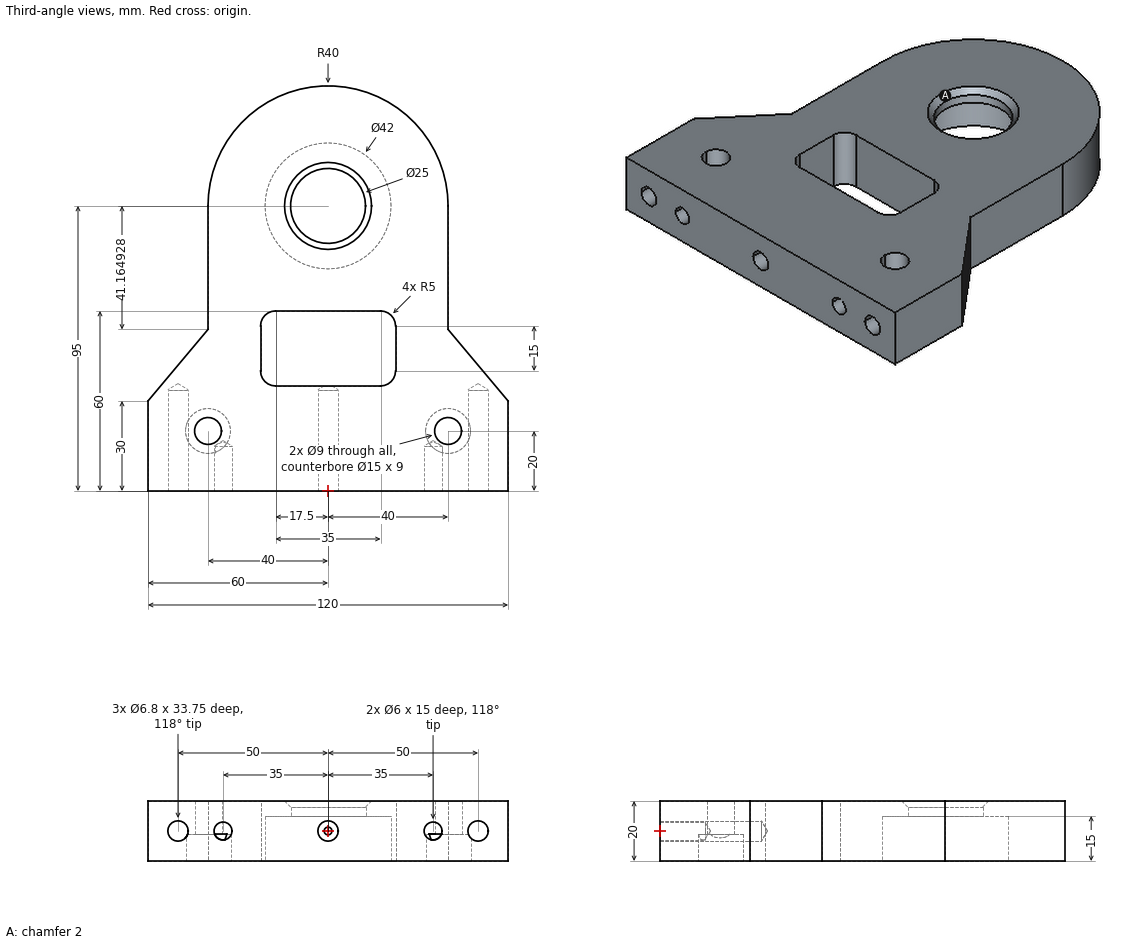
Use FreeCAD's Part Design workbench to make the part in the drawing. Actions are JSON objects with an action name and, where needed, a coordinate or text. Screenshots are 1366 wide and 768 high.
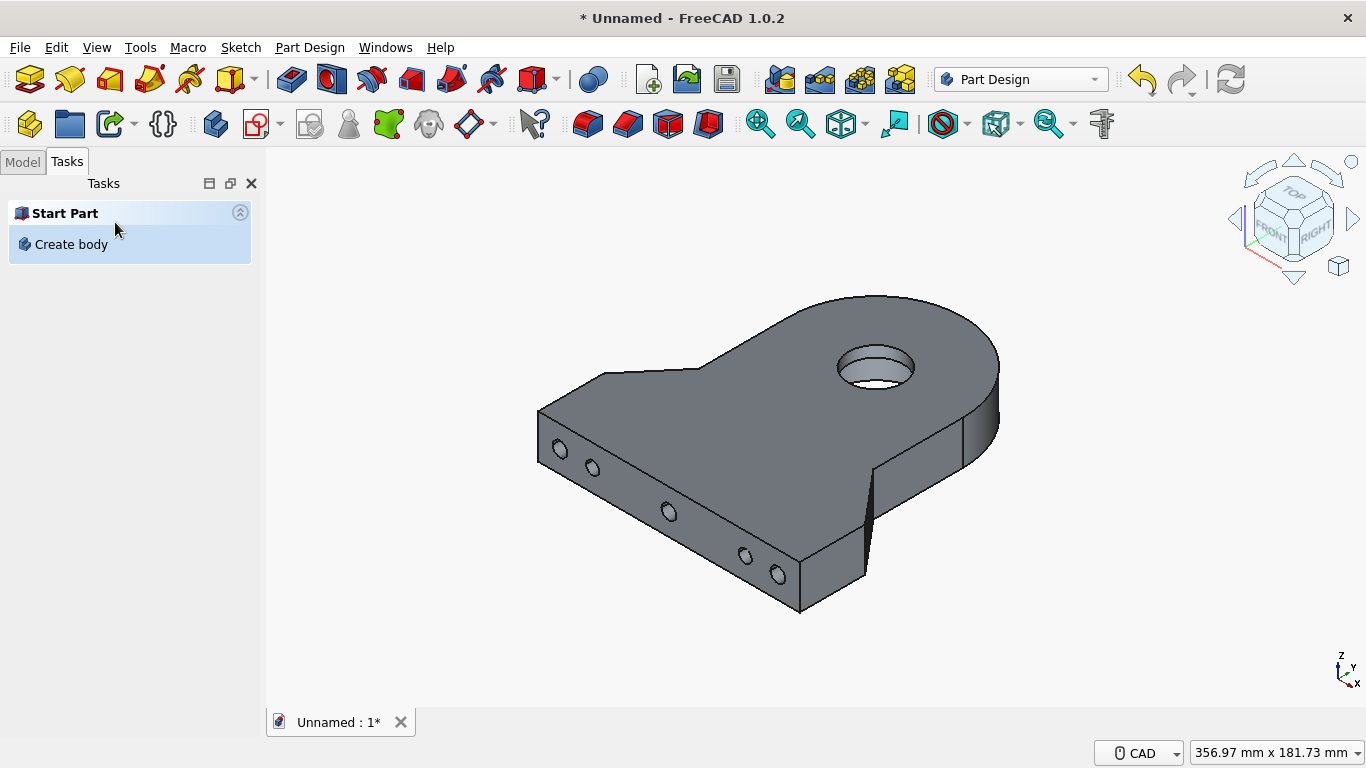
{"action": "left_click", "coordinate": [849, 351]}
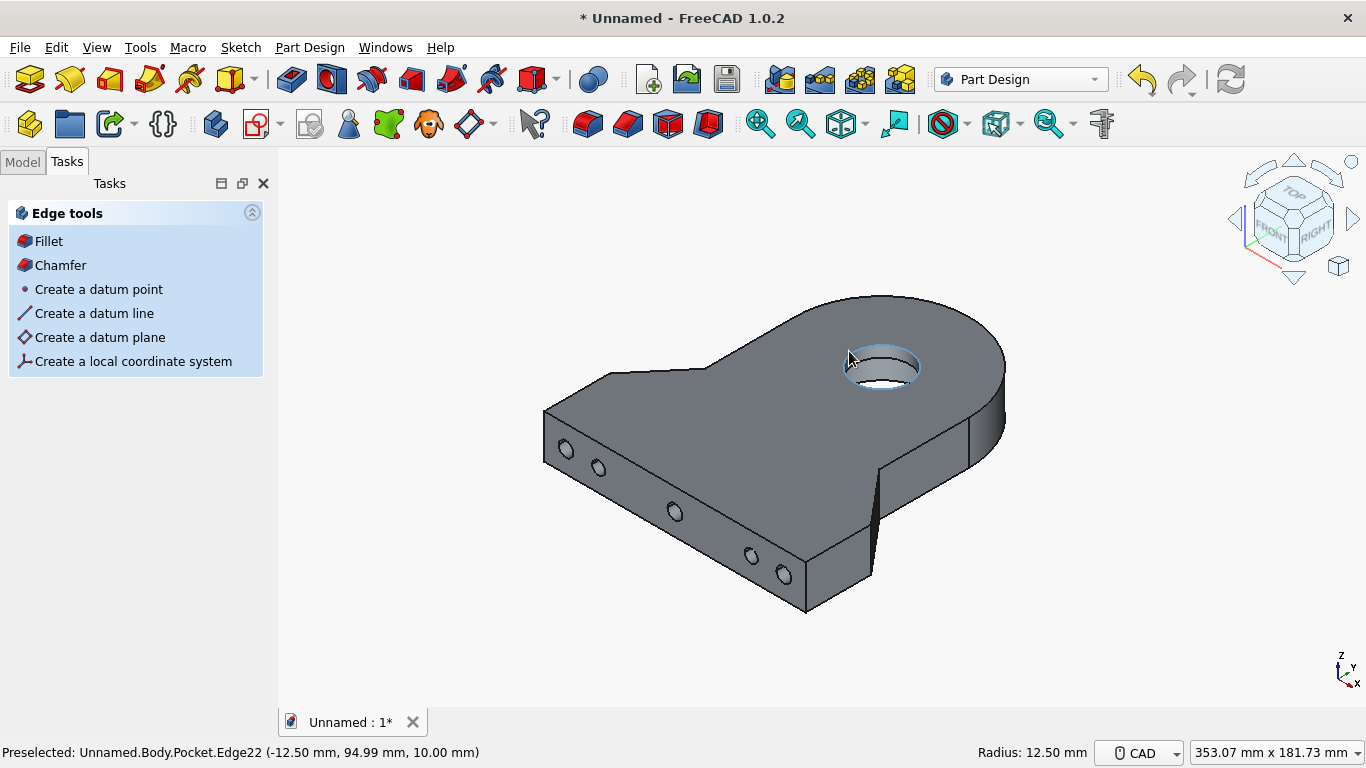
{"action": "left_click", "coordinate": [628, 124]}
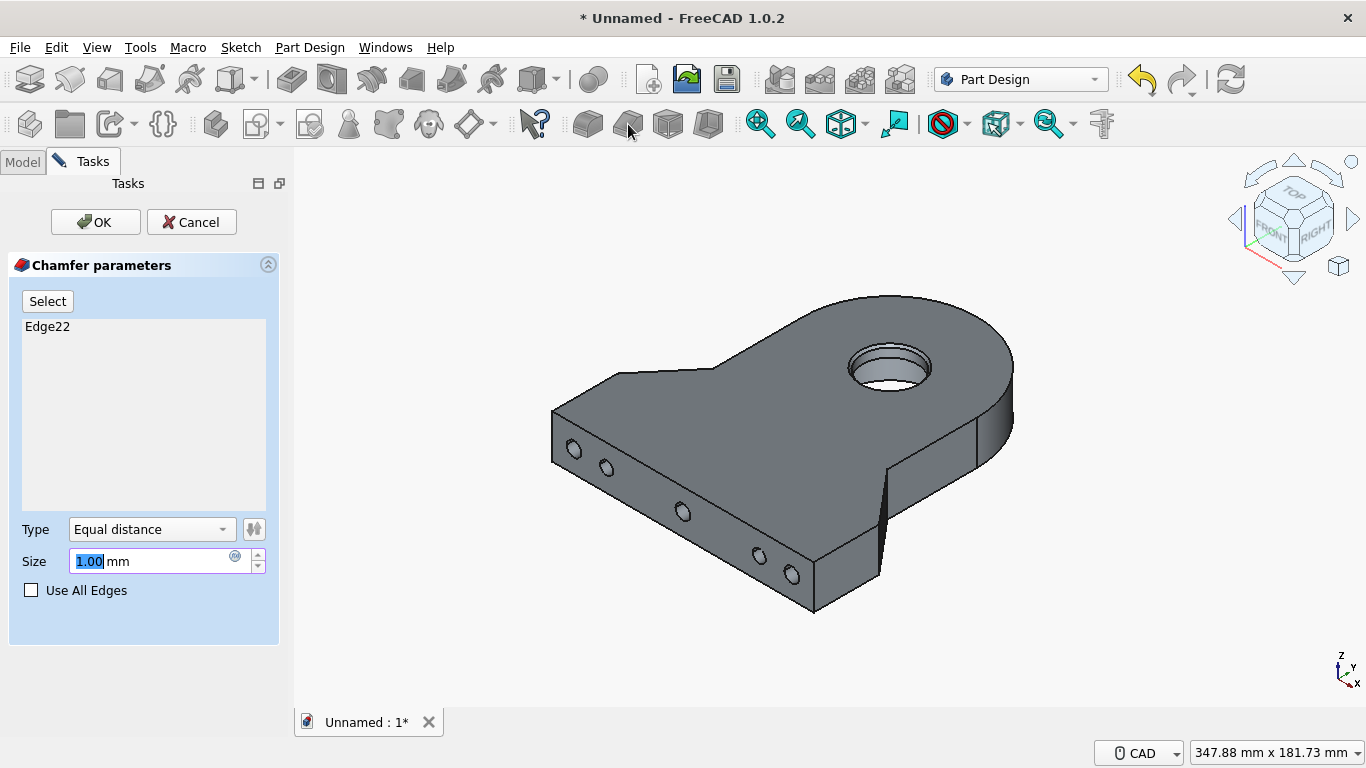
{"action": "type", "text": "2"}
{"action": "key", "text": "Tab"}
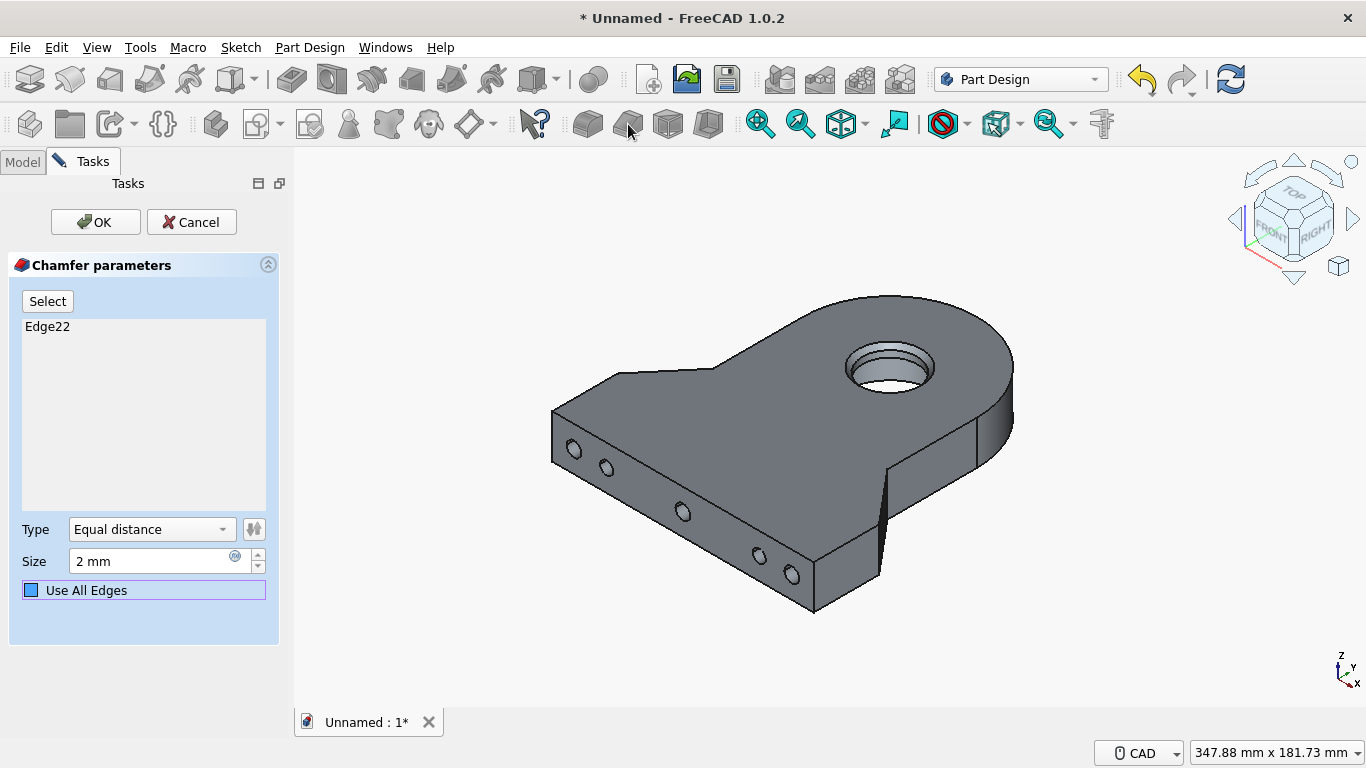
{"action": "left_click", "coordinate": [96, 222]}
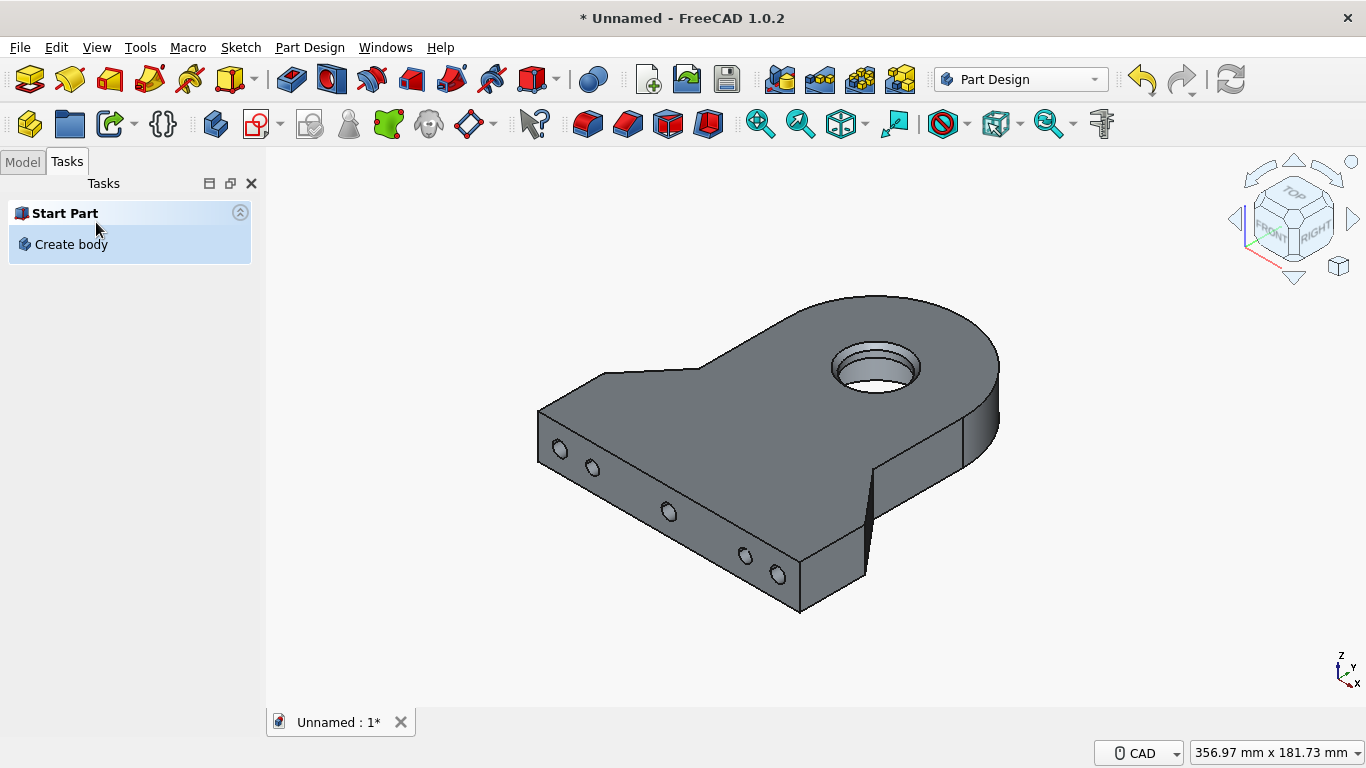
{"action": "key", "text": "5"}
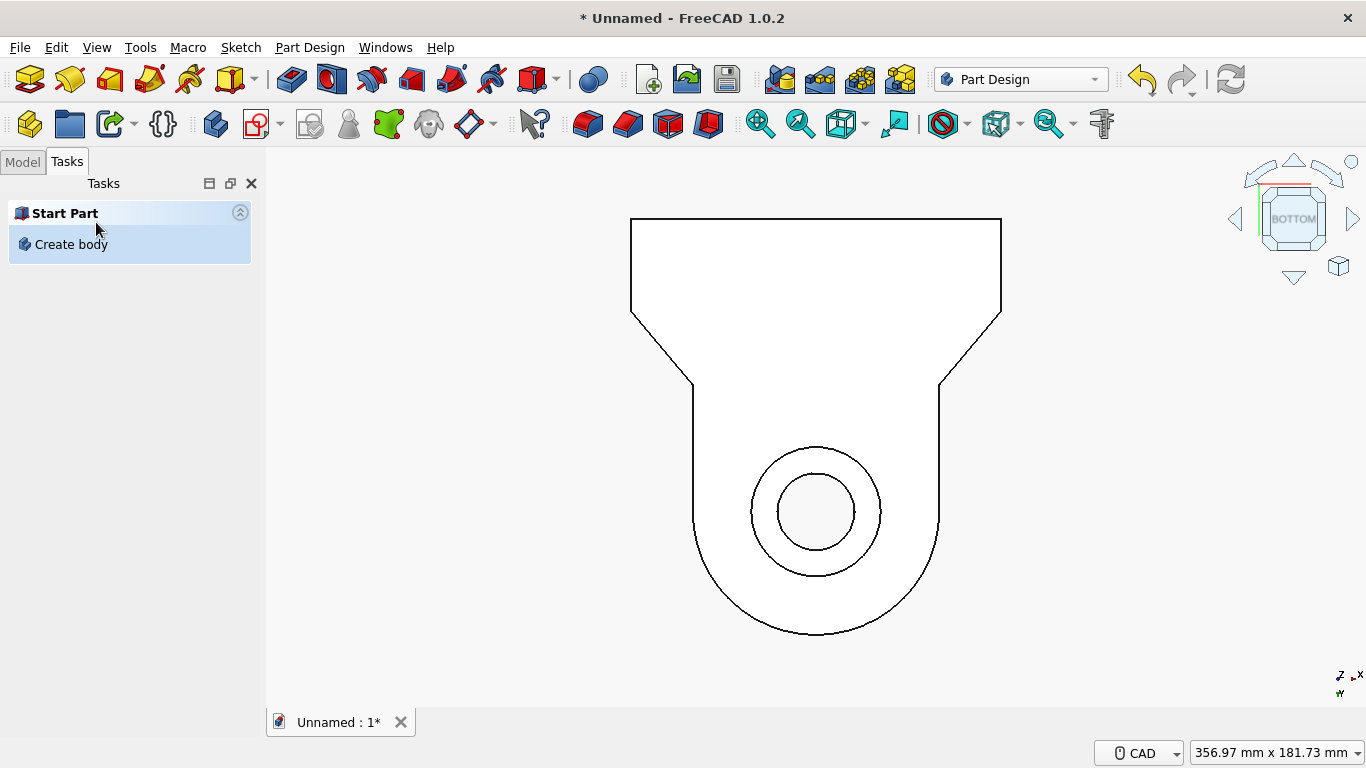
{"action": "left_click", "coordinate": [869, 307]}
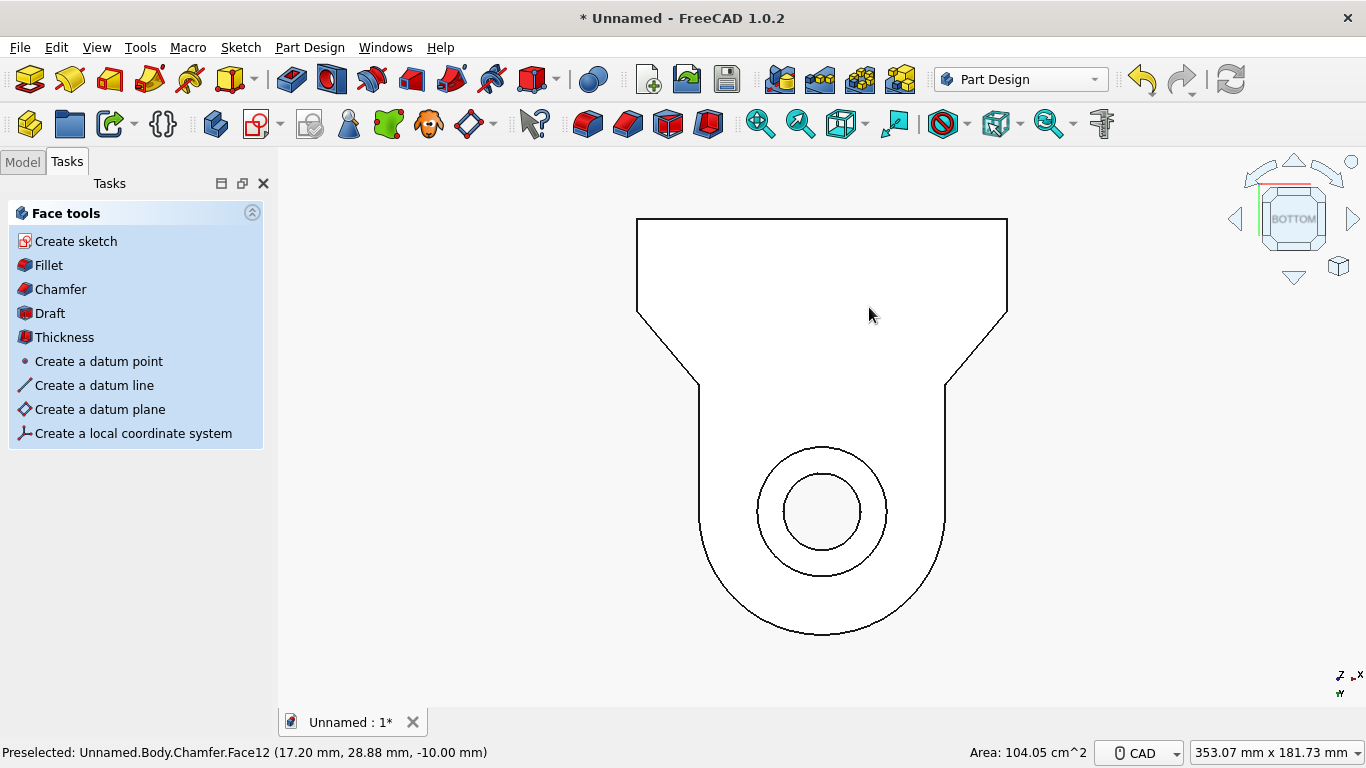
{"action": "left_click", "coordinate": [256, 124]}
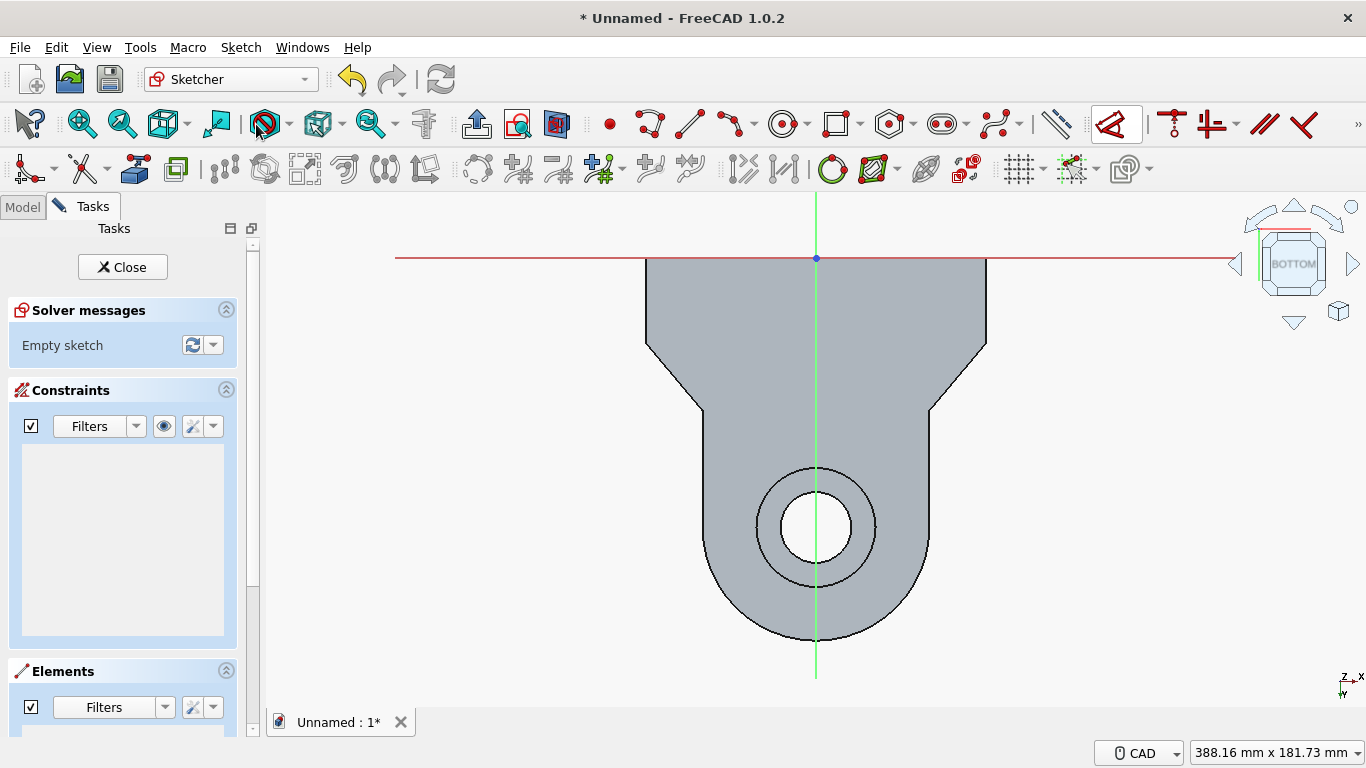
{"action": "scroll", "coordinate": [856, 220], "scroll_direction": "up", "scroll_amount": 5}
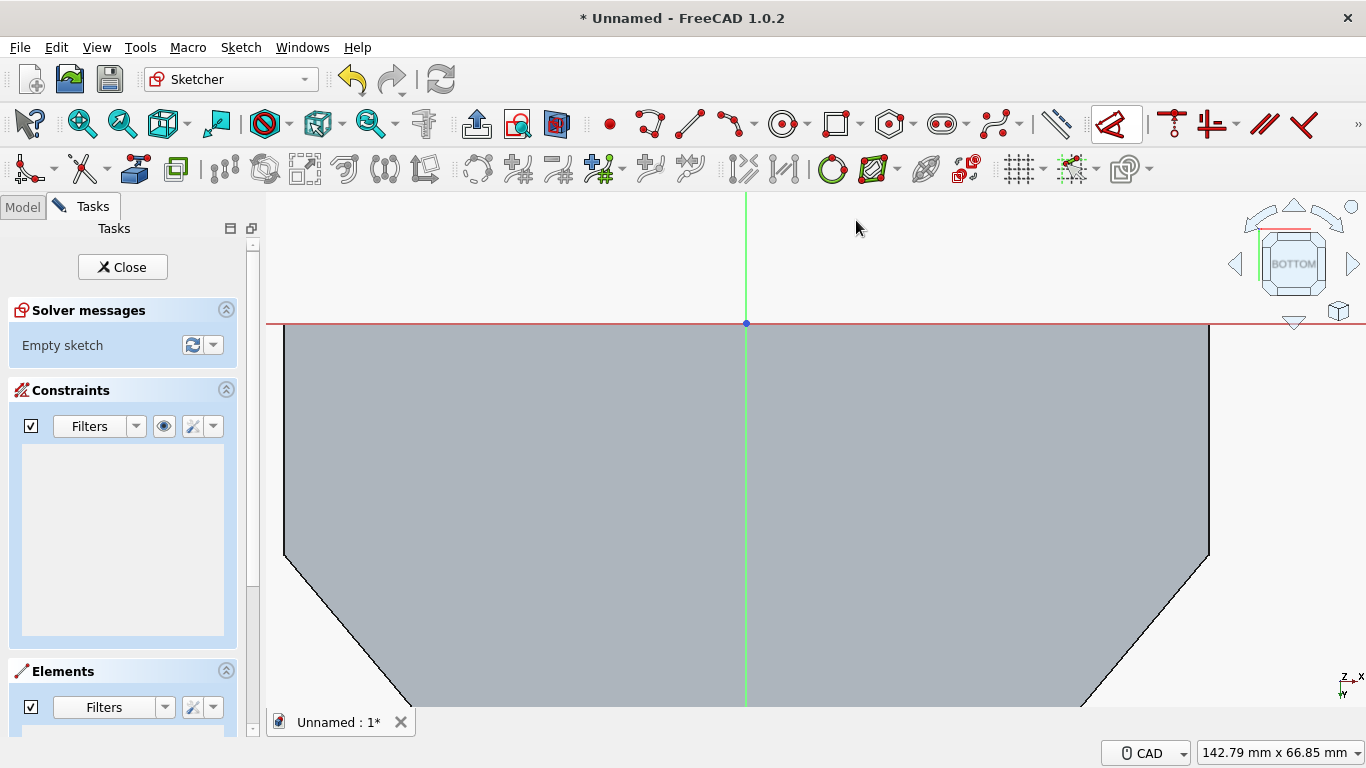
{"action": "left_click", "coordinate": [784, 124]}